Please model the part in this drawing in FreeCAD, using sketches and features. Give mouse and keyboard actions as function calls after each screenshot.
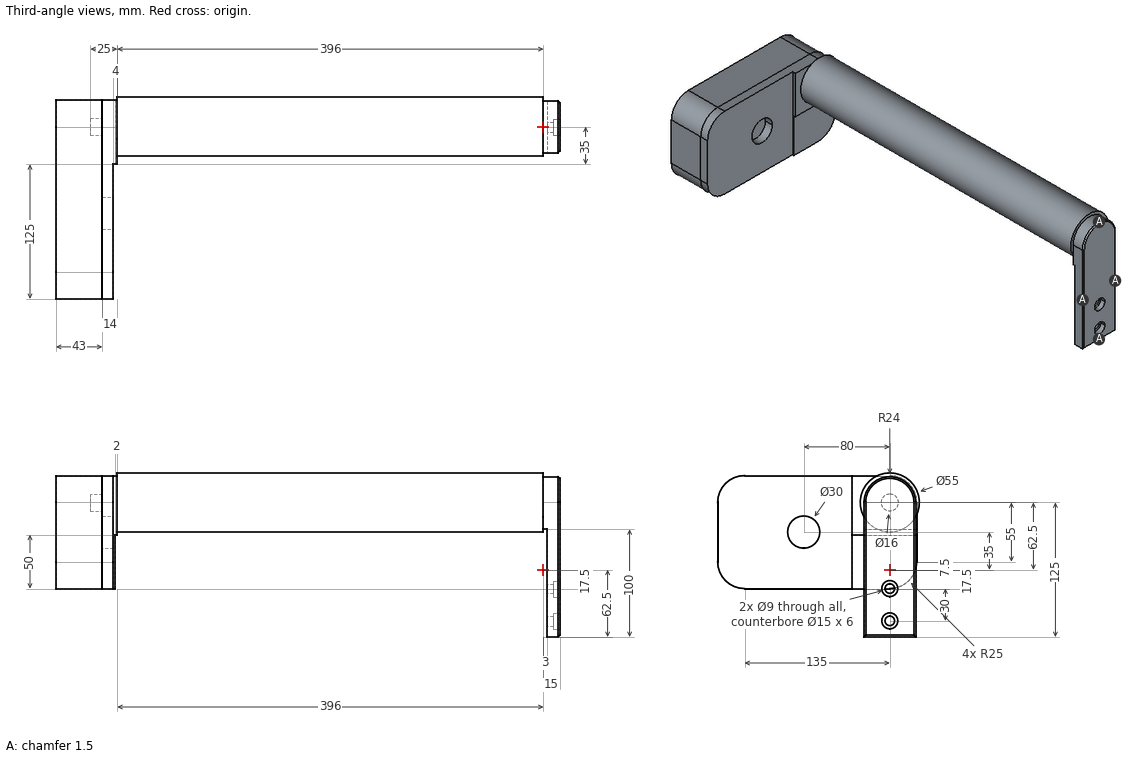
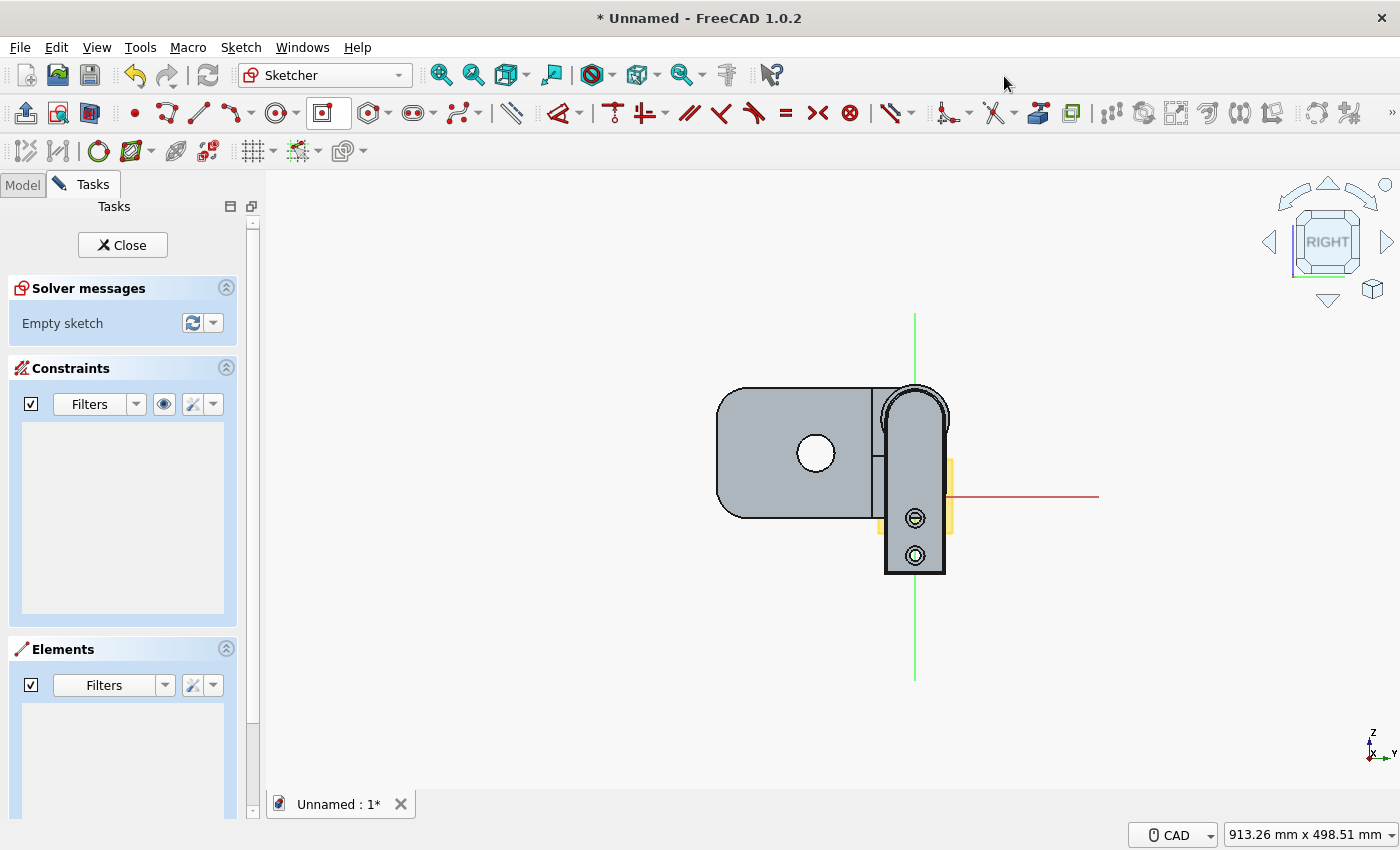
scroll(870, 438, up, 5)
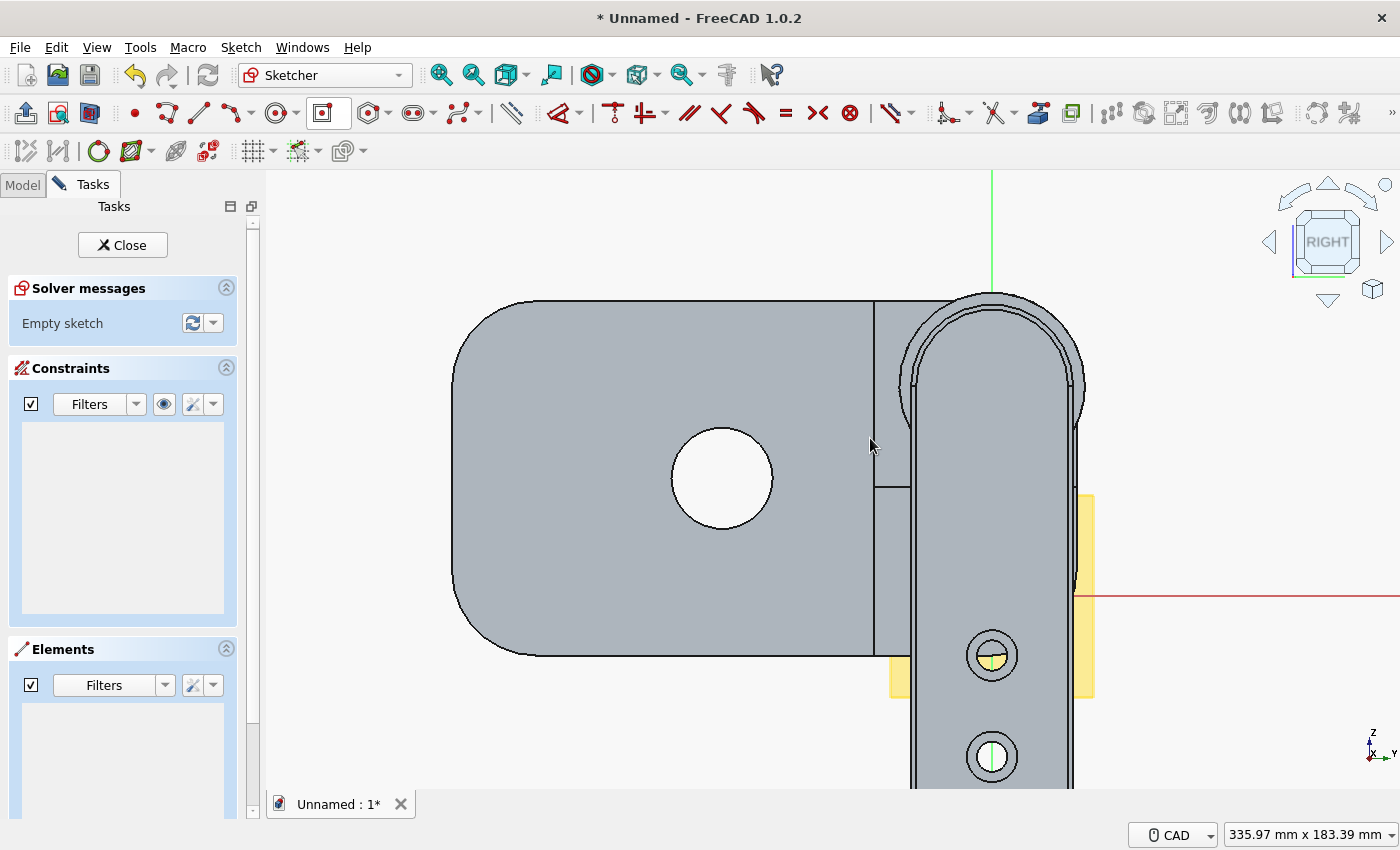
key(g)
key(l)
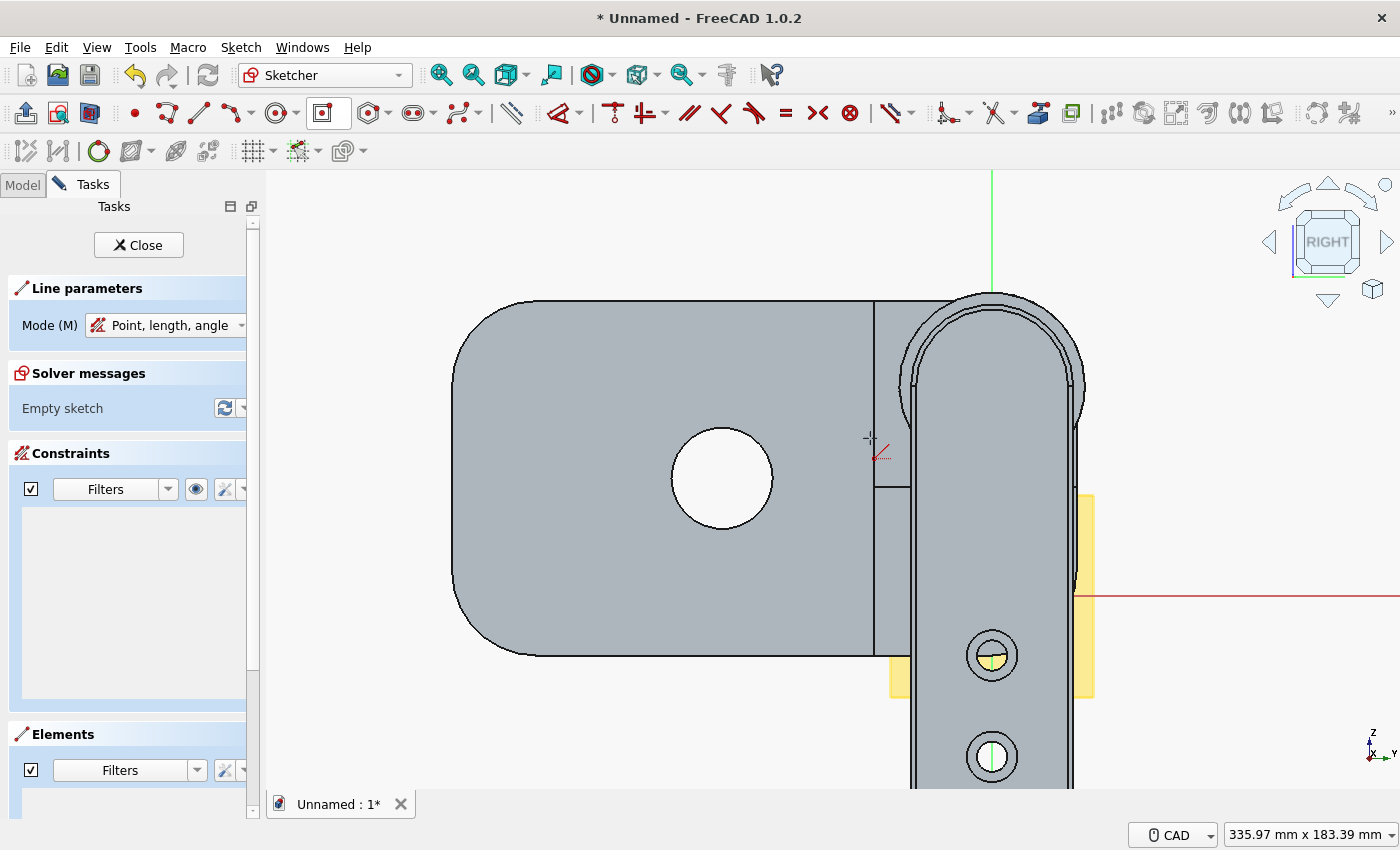
click(1077, 386)
click(1077, 571)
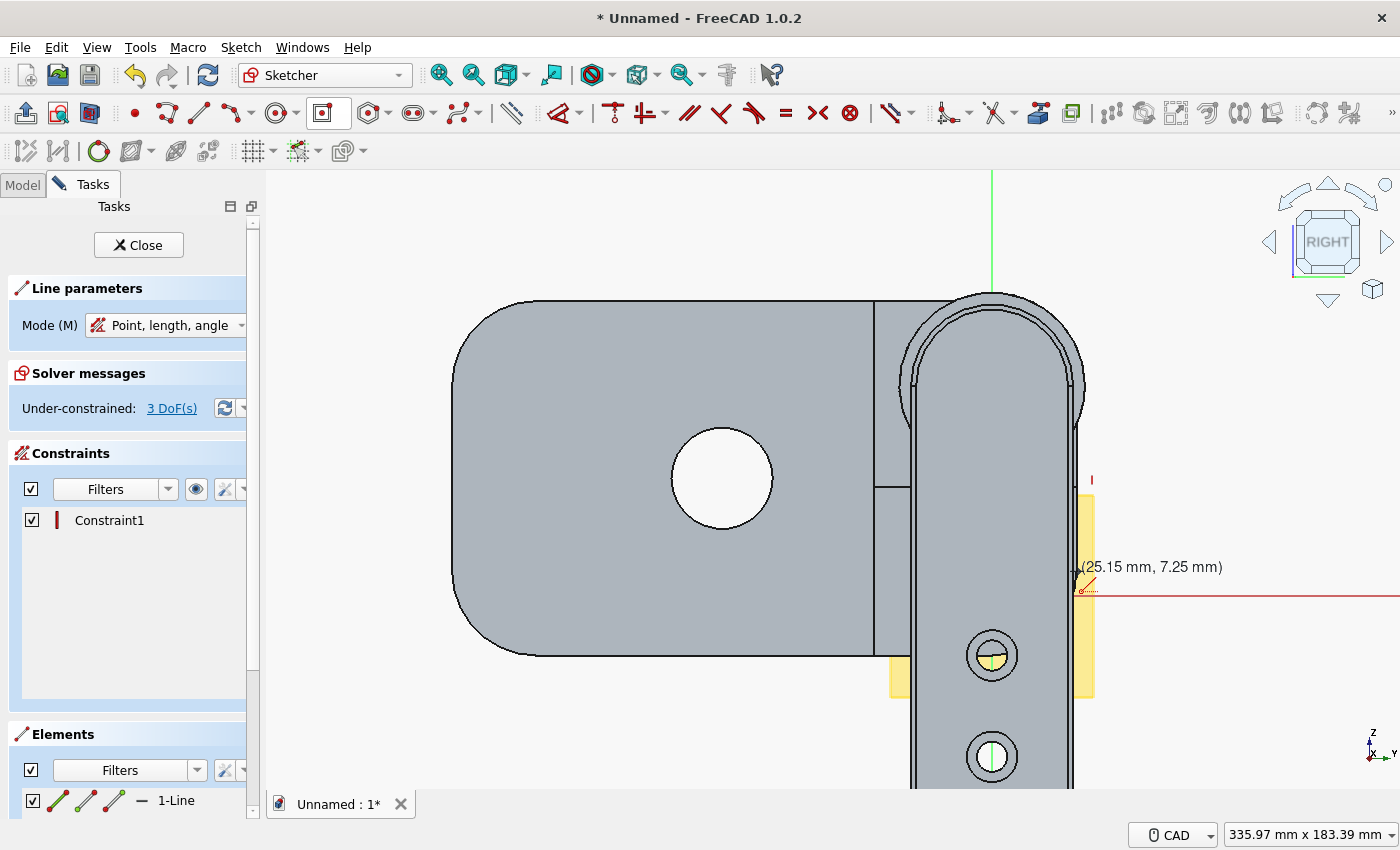
click(992, 656)
click(536, 656)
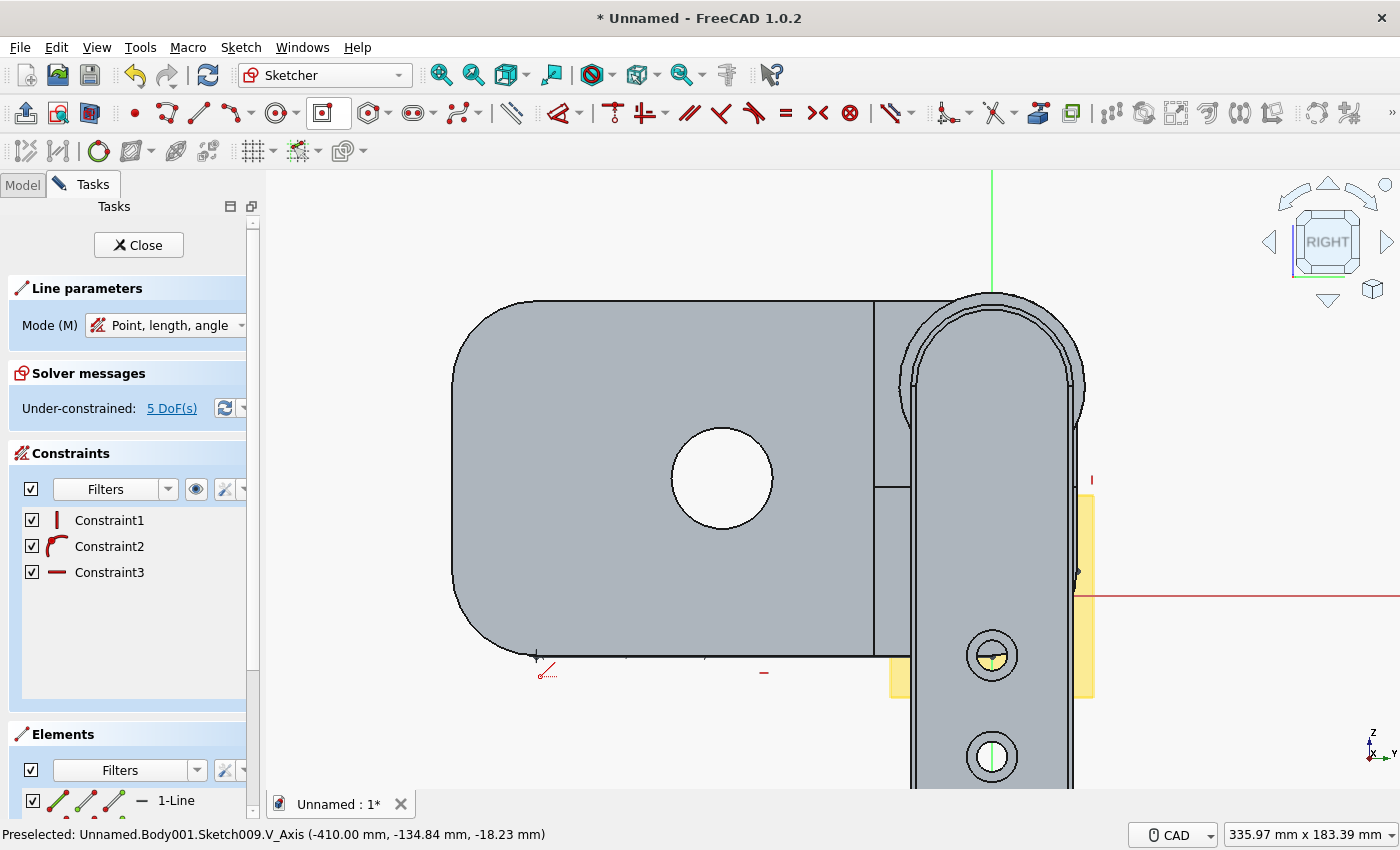
click(452, 571)
click(452, 386)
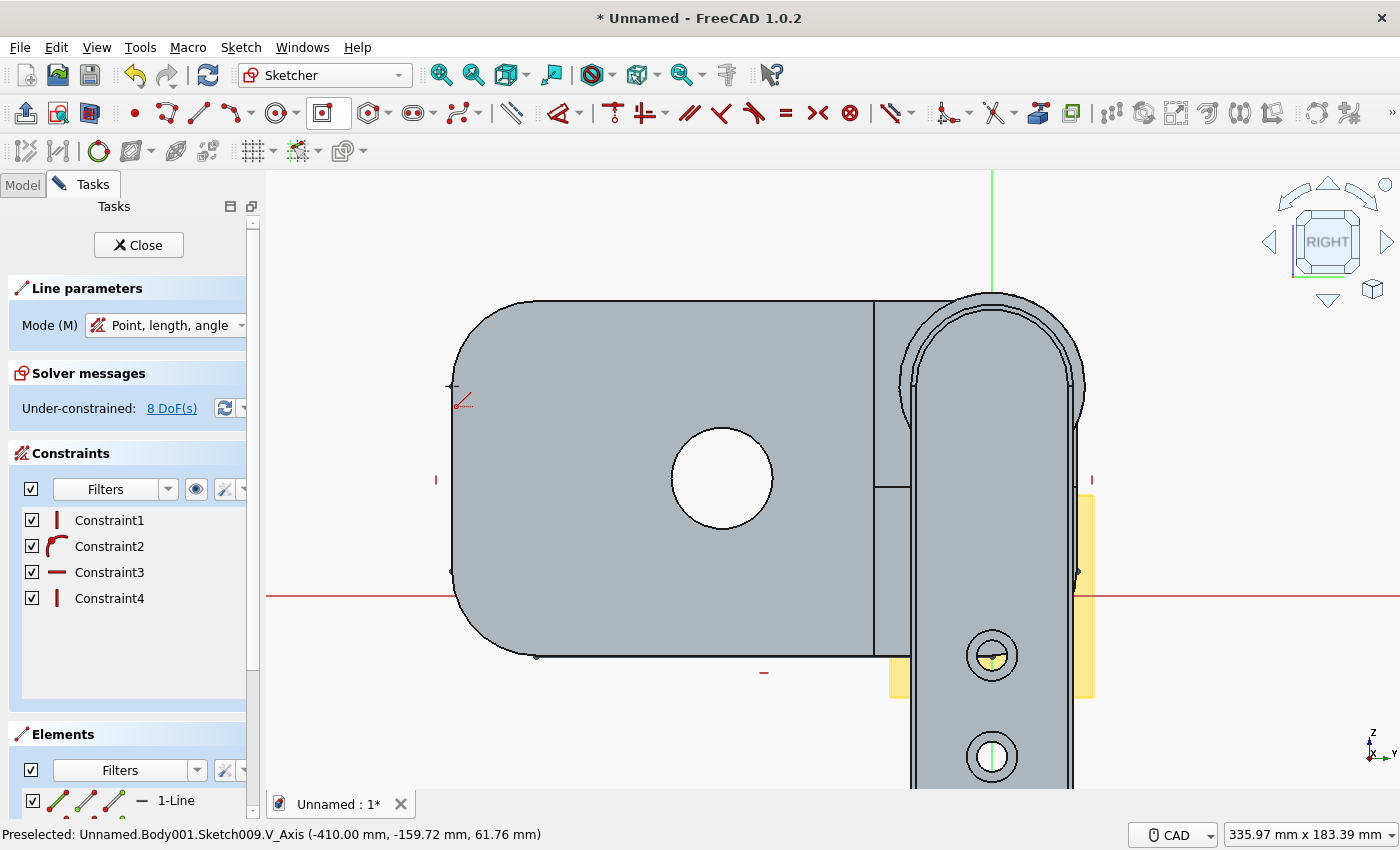
click(536, 301)
click(992, 301)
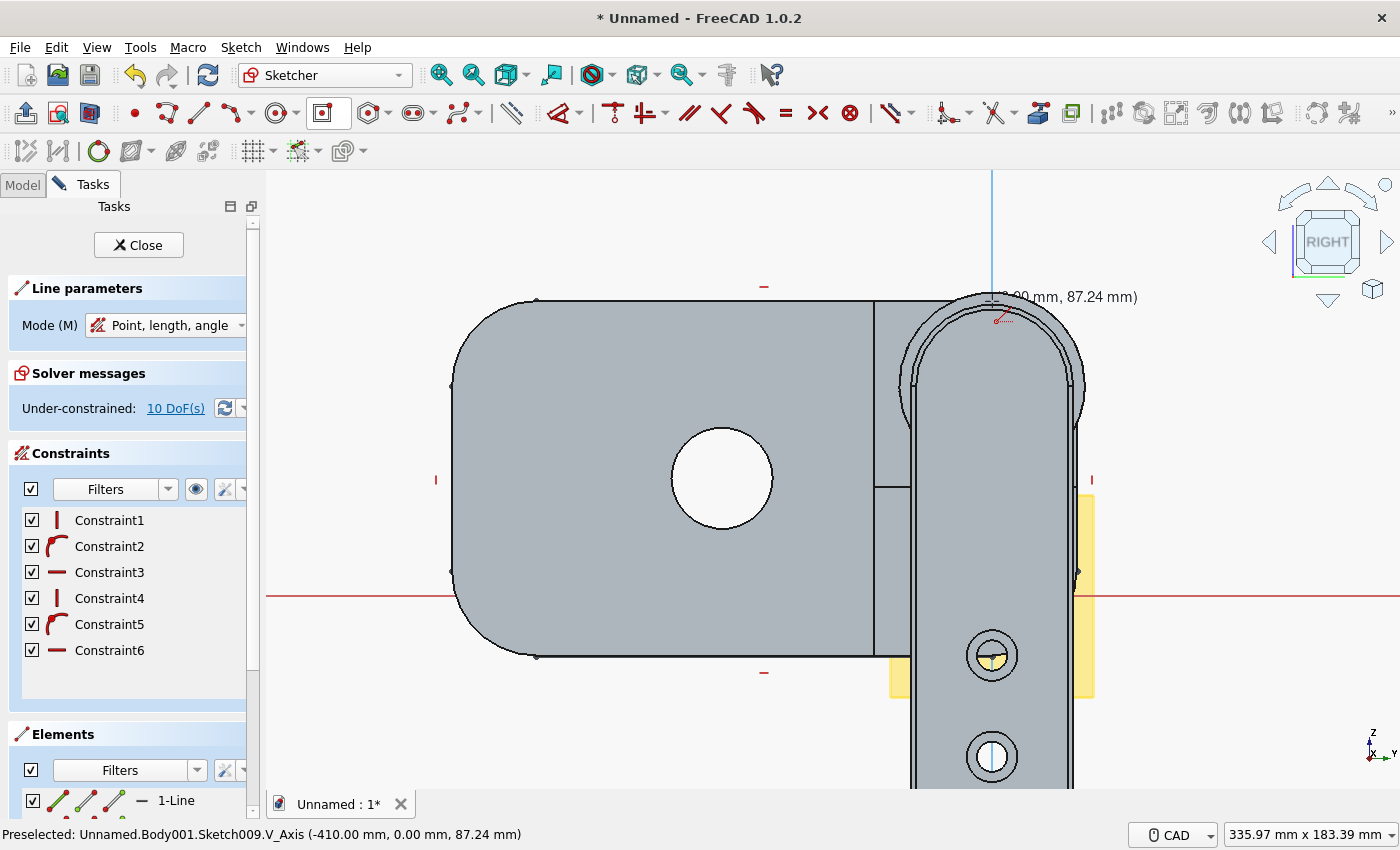
click(232, 114)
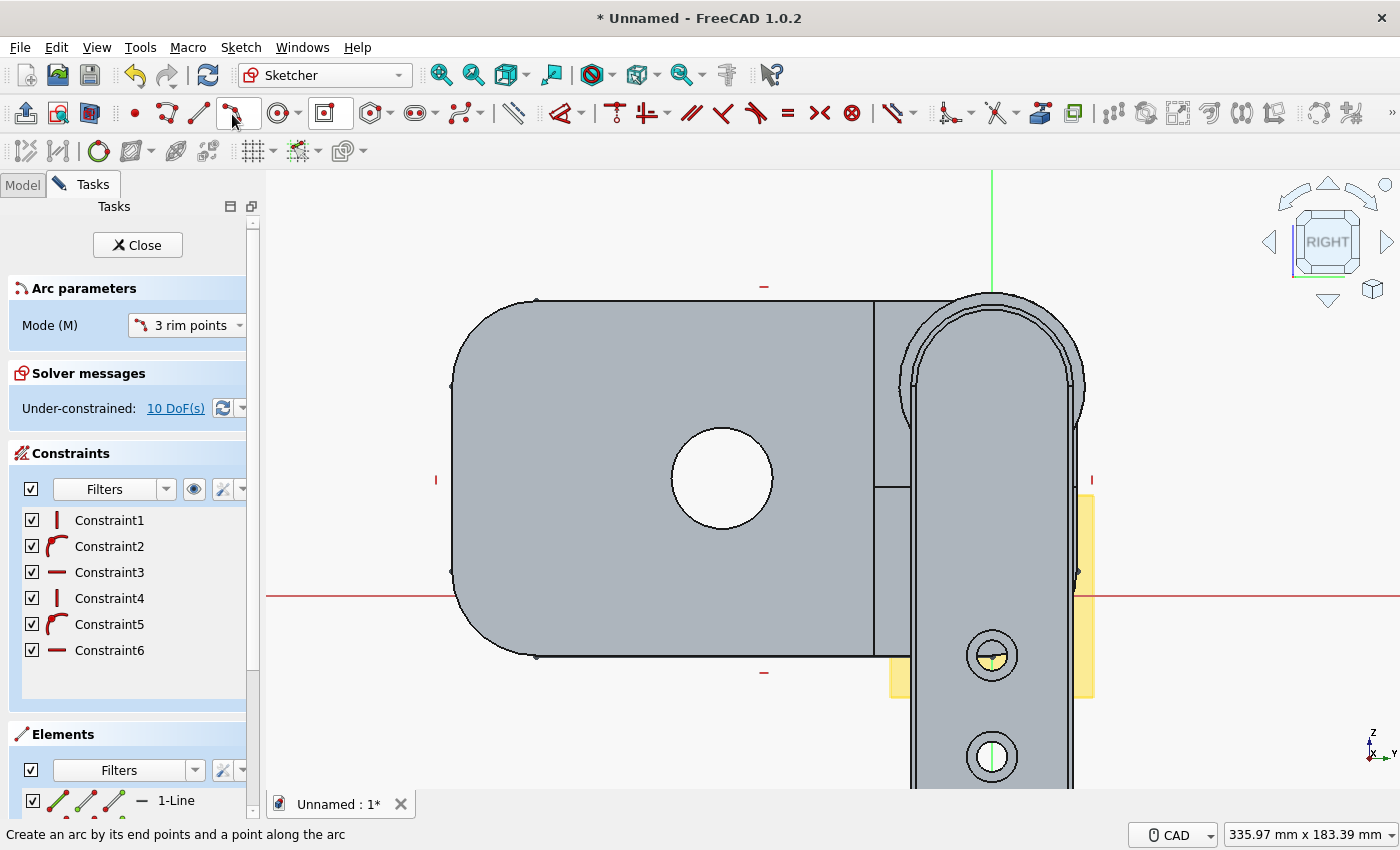
click(1077, 572)
click(992, 657)
click(1052, 631)